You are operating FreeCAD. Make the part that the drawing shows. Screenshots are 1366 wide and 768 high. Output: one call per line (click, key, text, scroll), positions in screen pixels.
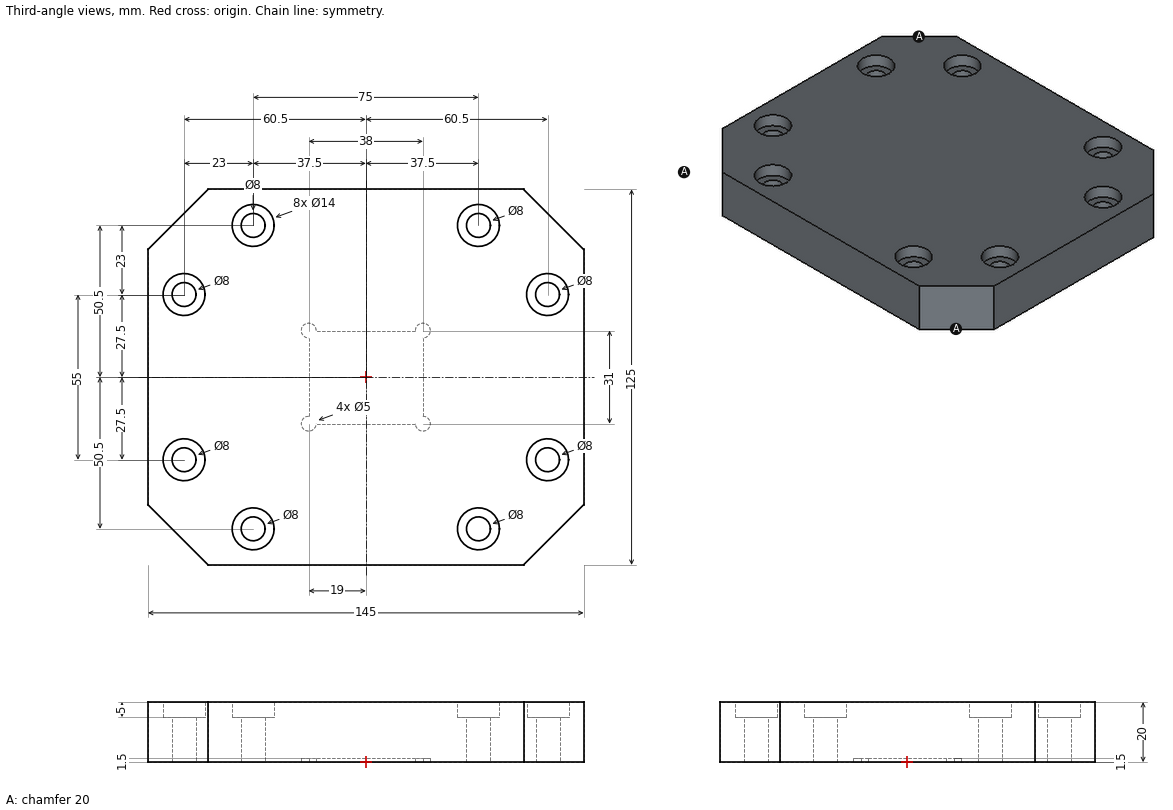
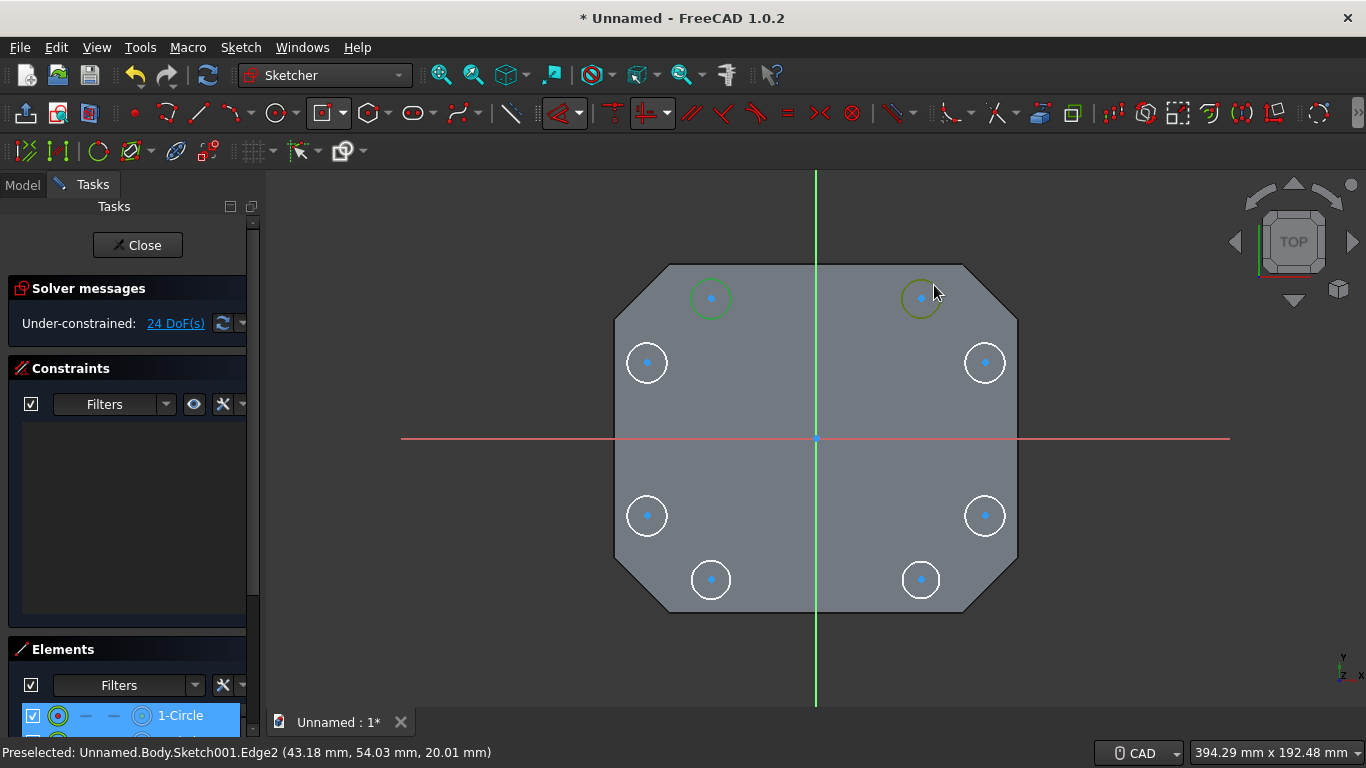
click(661, 349)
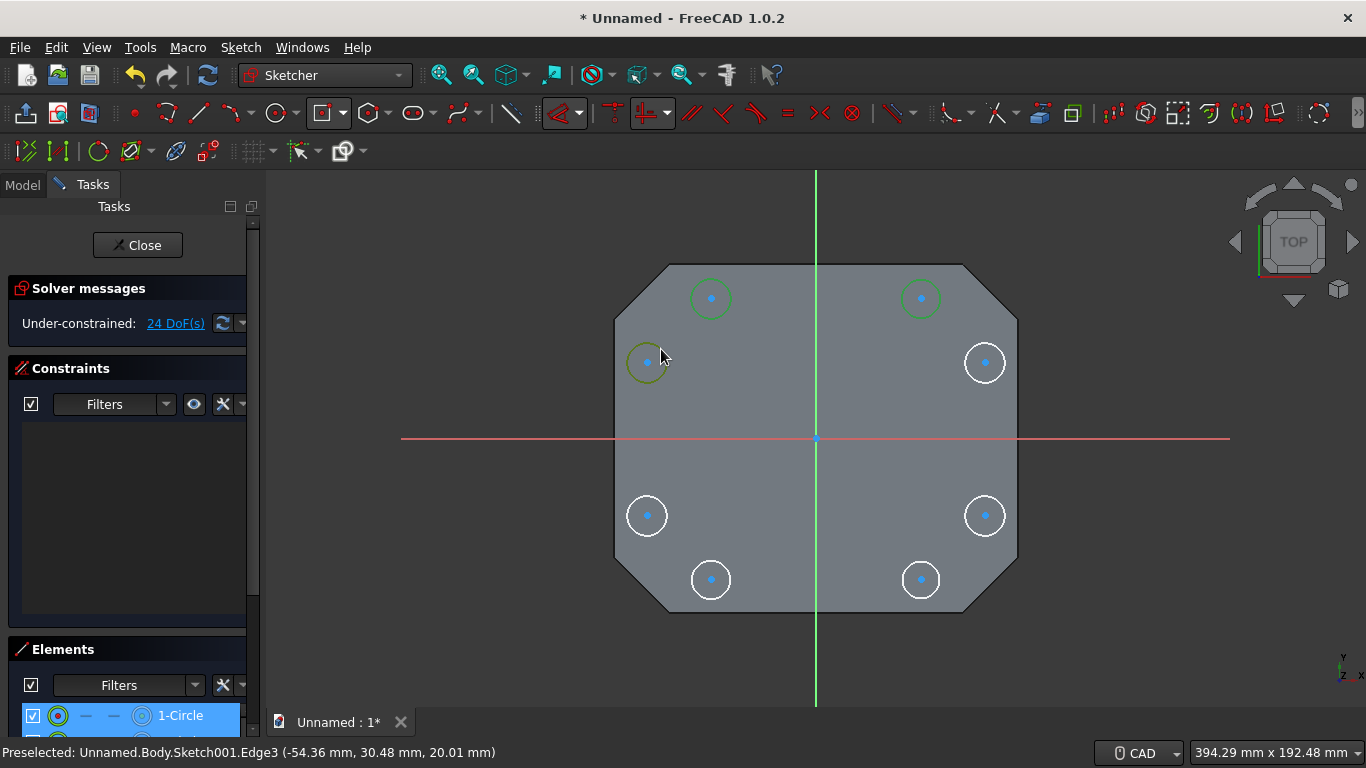
click(661, 502)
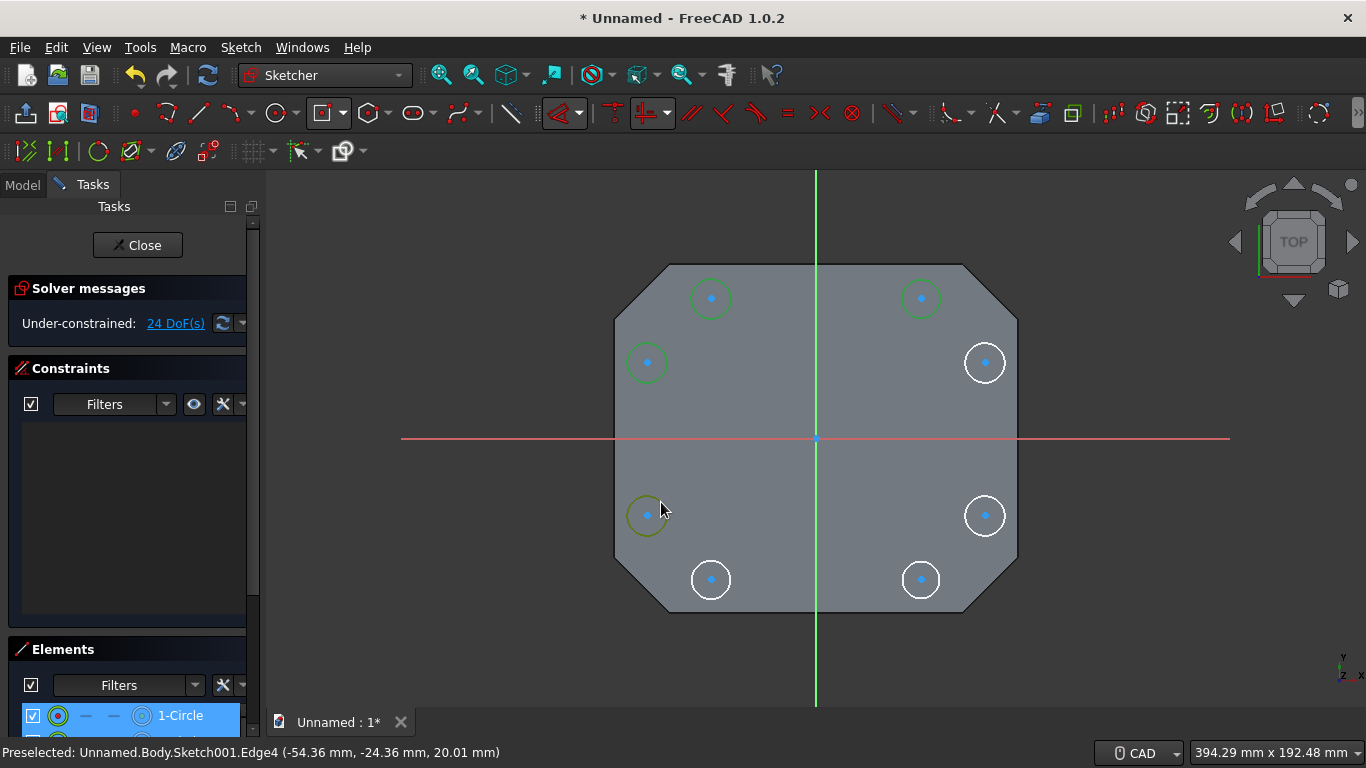
click(724, 566)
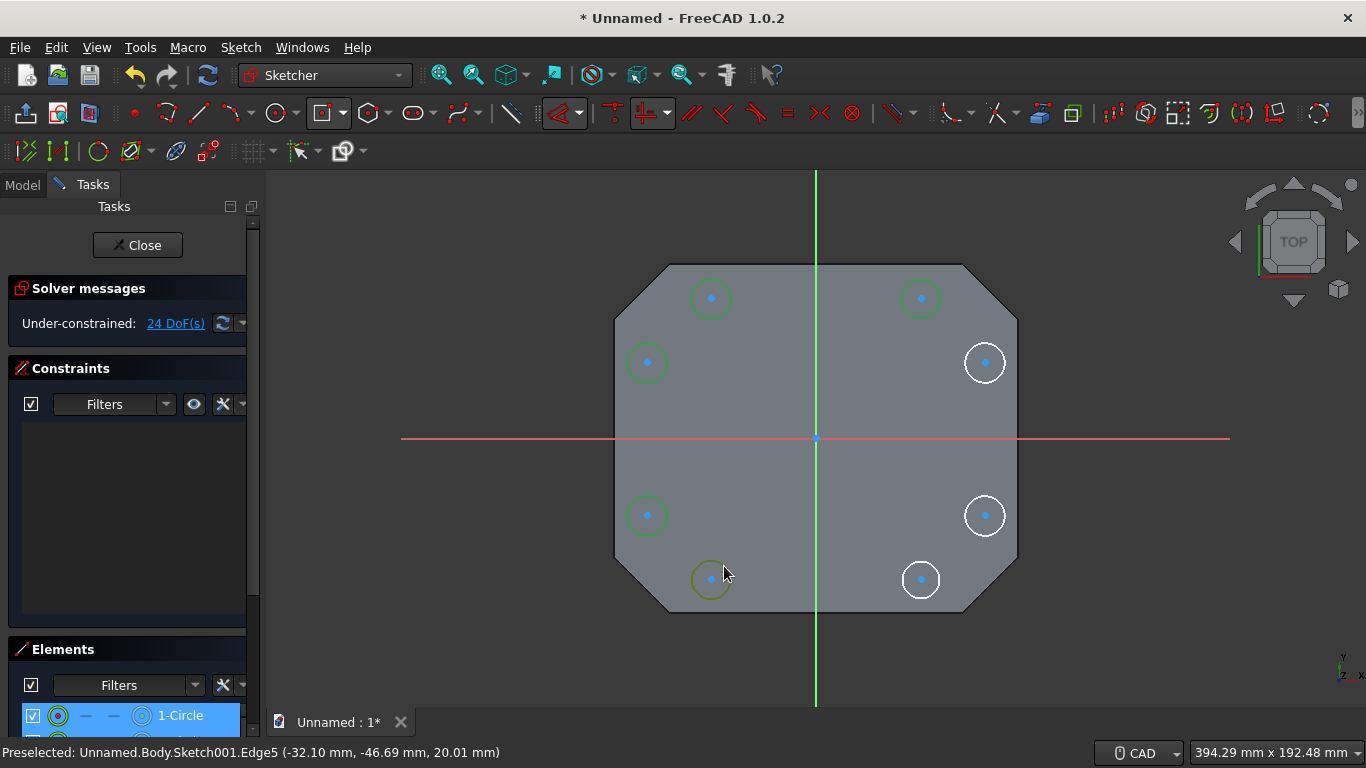
click(934, 567)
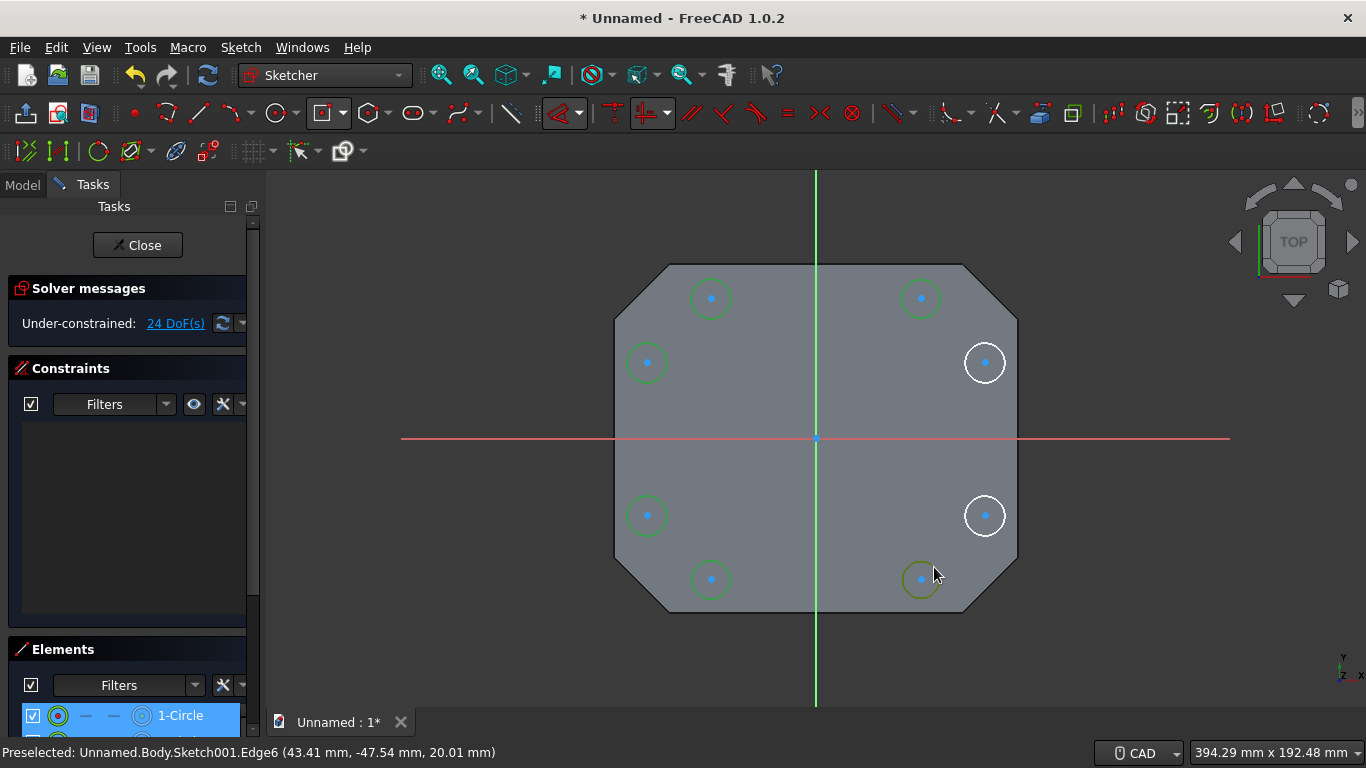
click(999, 349)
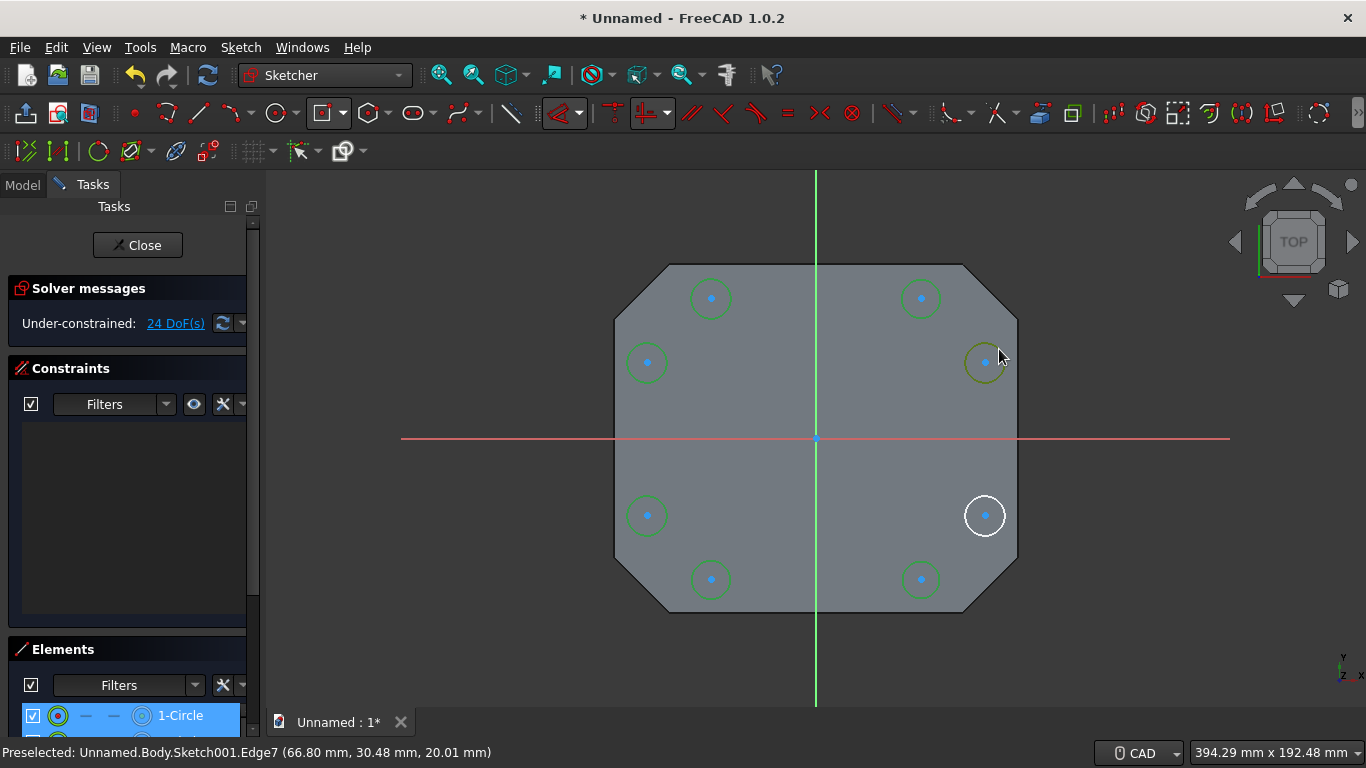
click(999, 502)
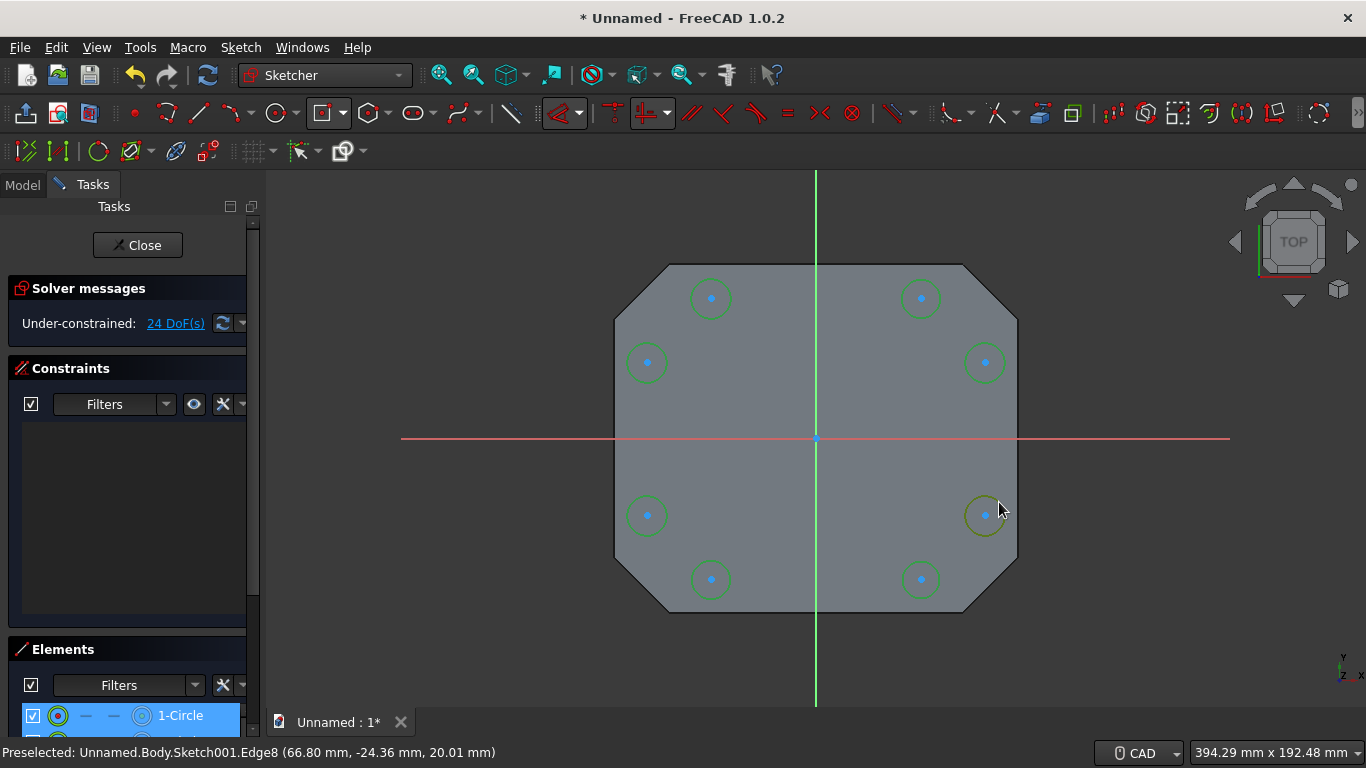
key(e)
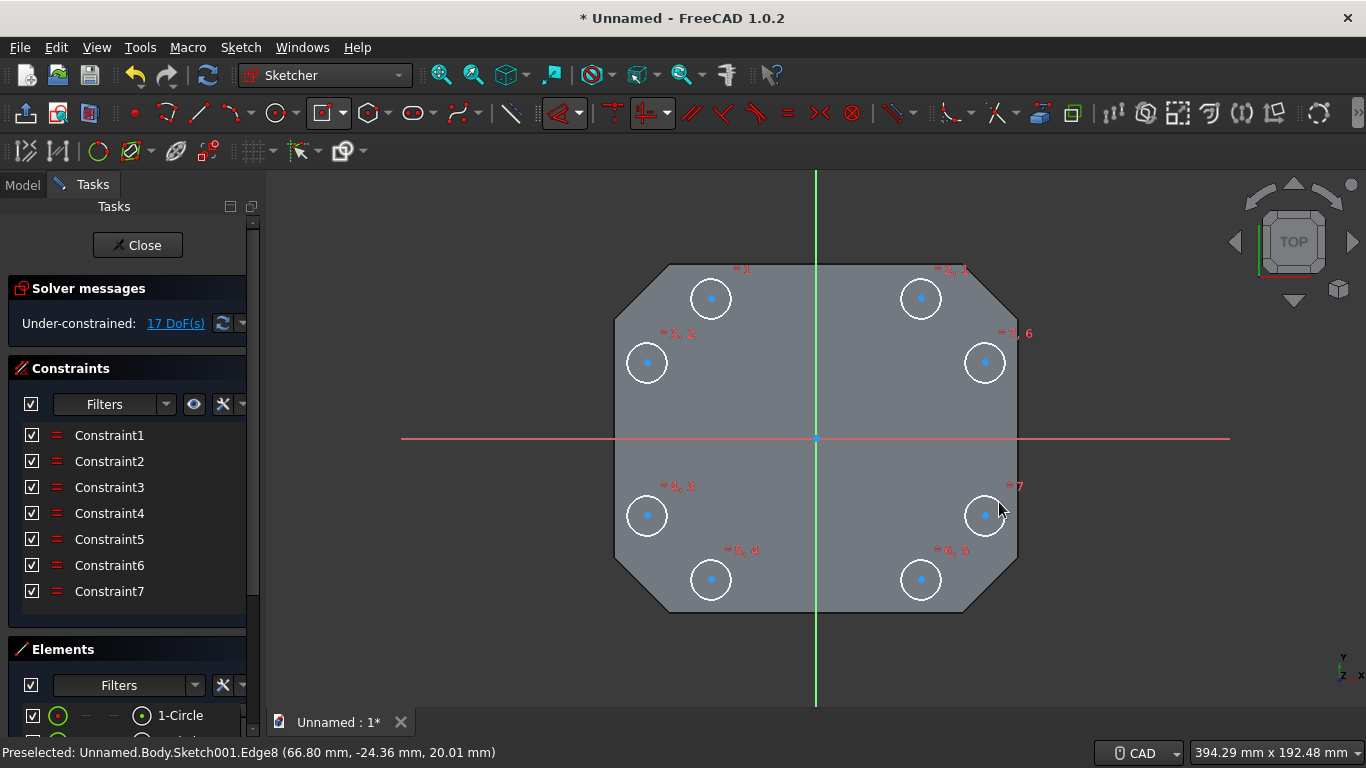
click(711, 299)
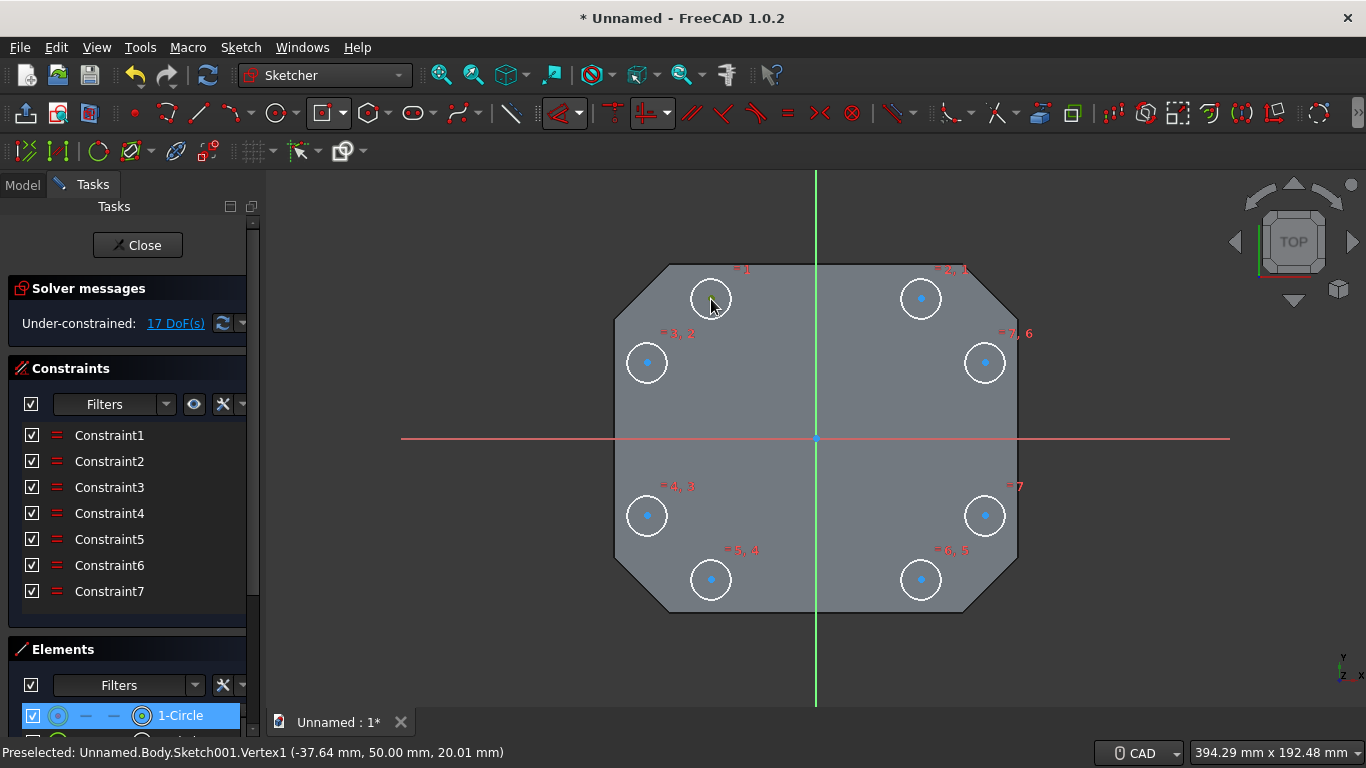
click(921, 299)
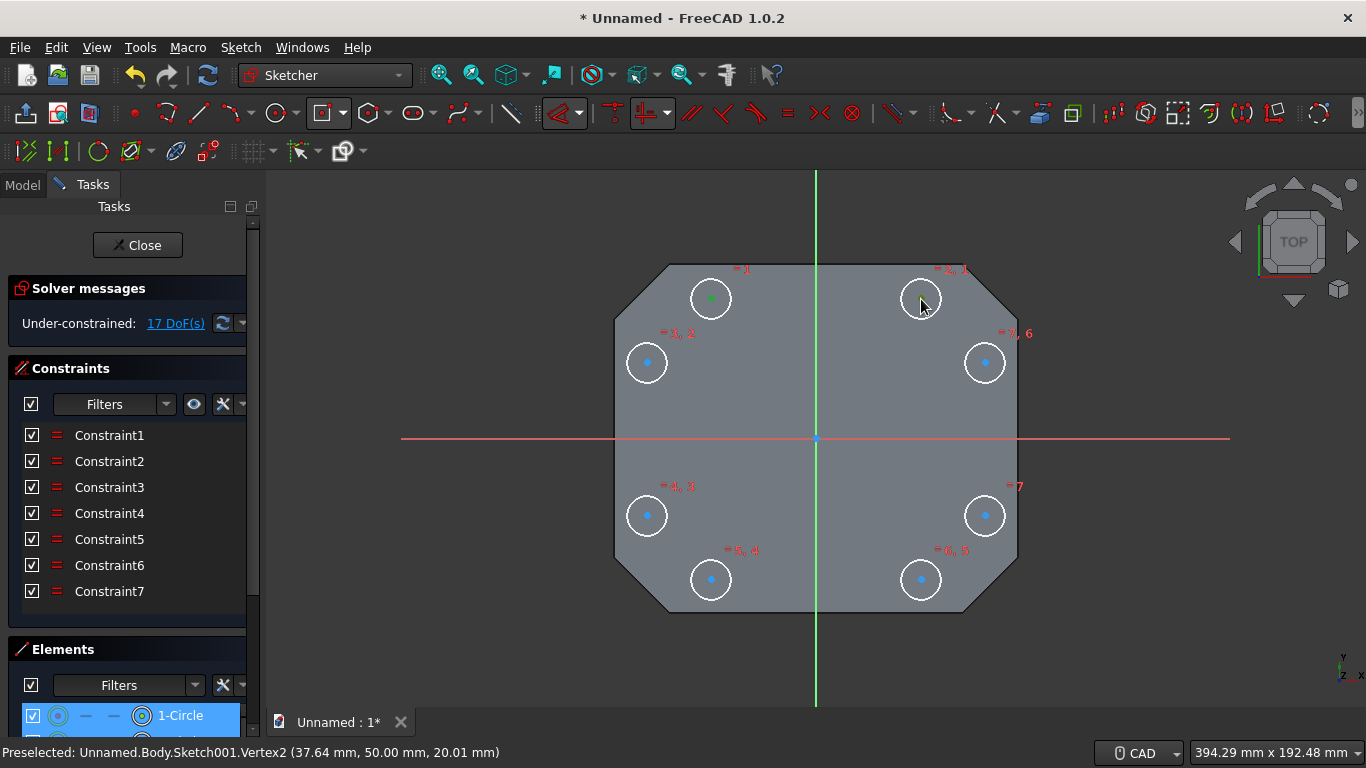
click(816, 645)